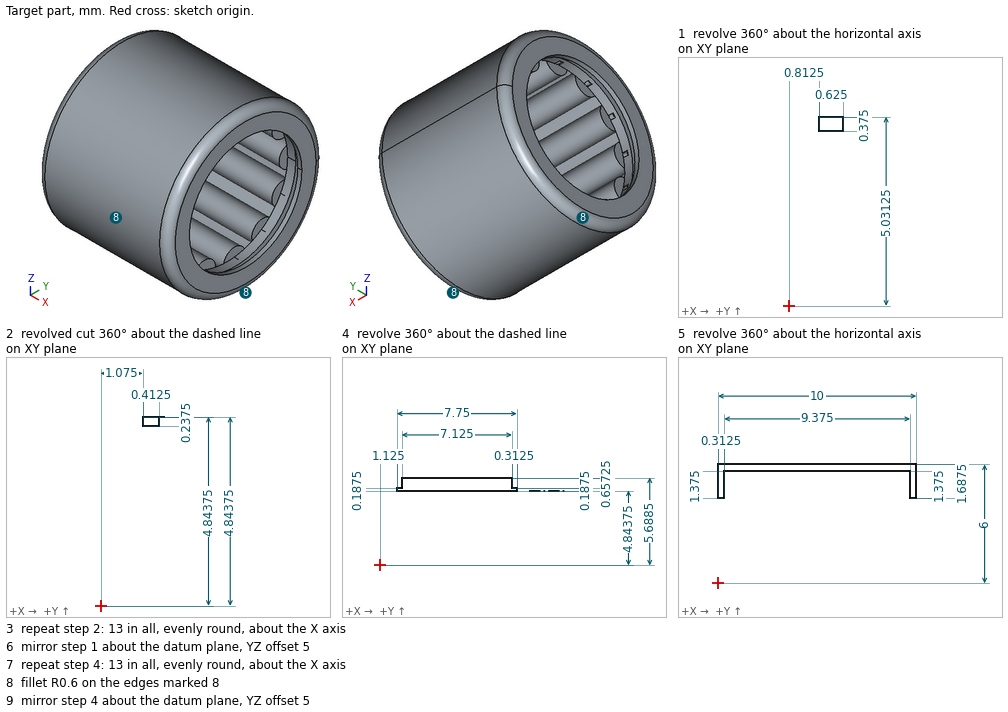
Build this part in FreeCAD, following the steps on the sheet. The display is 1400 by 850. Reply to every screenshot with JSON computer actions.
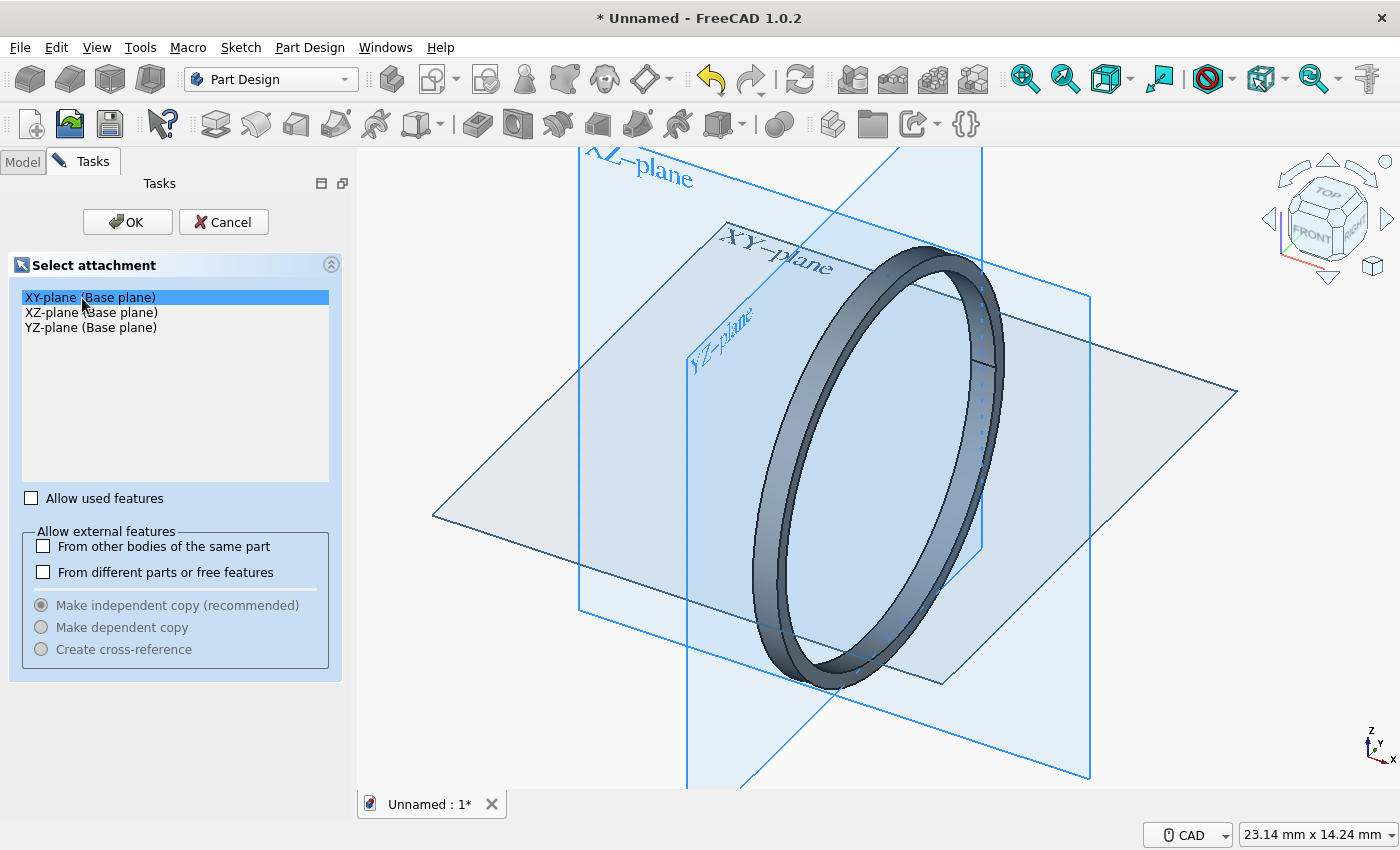
{"action": "left_click", "coordinate": [128, 222]}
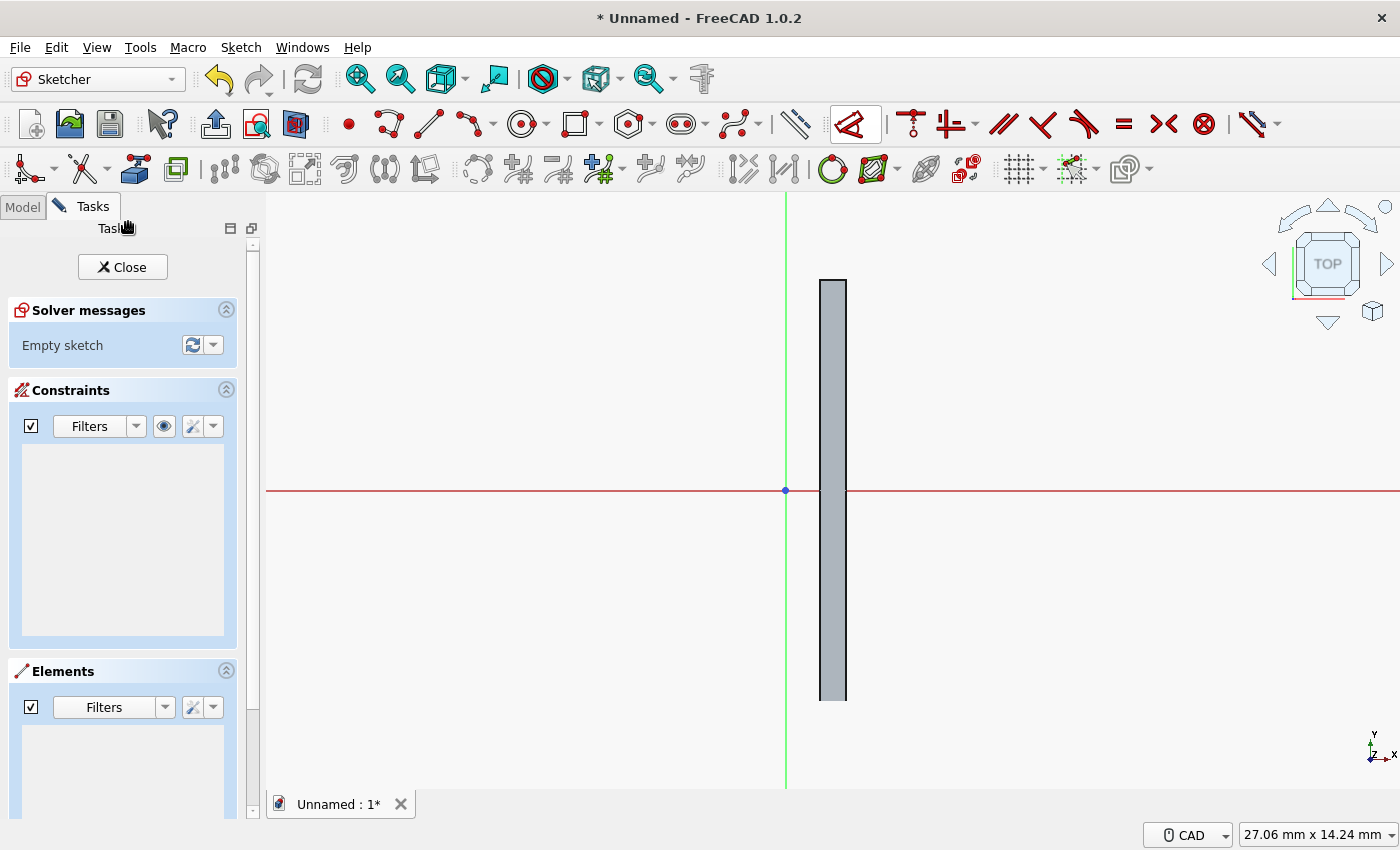
{"action": "key", "text": "q s"}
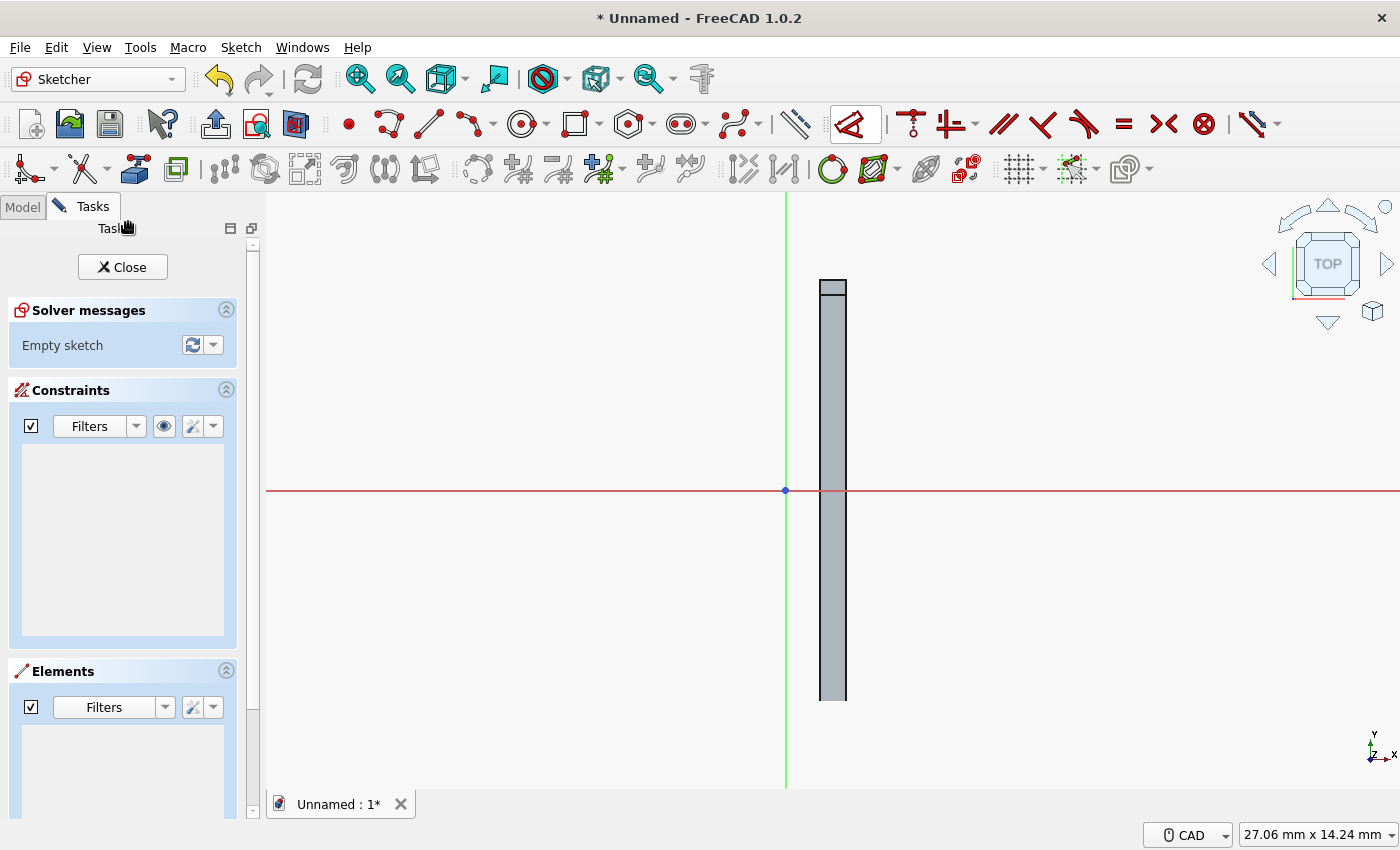
{"action": "scroll", "coordinate": [847, 282], "scroll_direction": "up", "scroll_amount": 15}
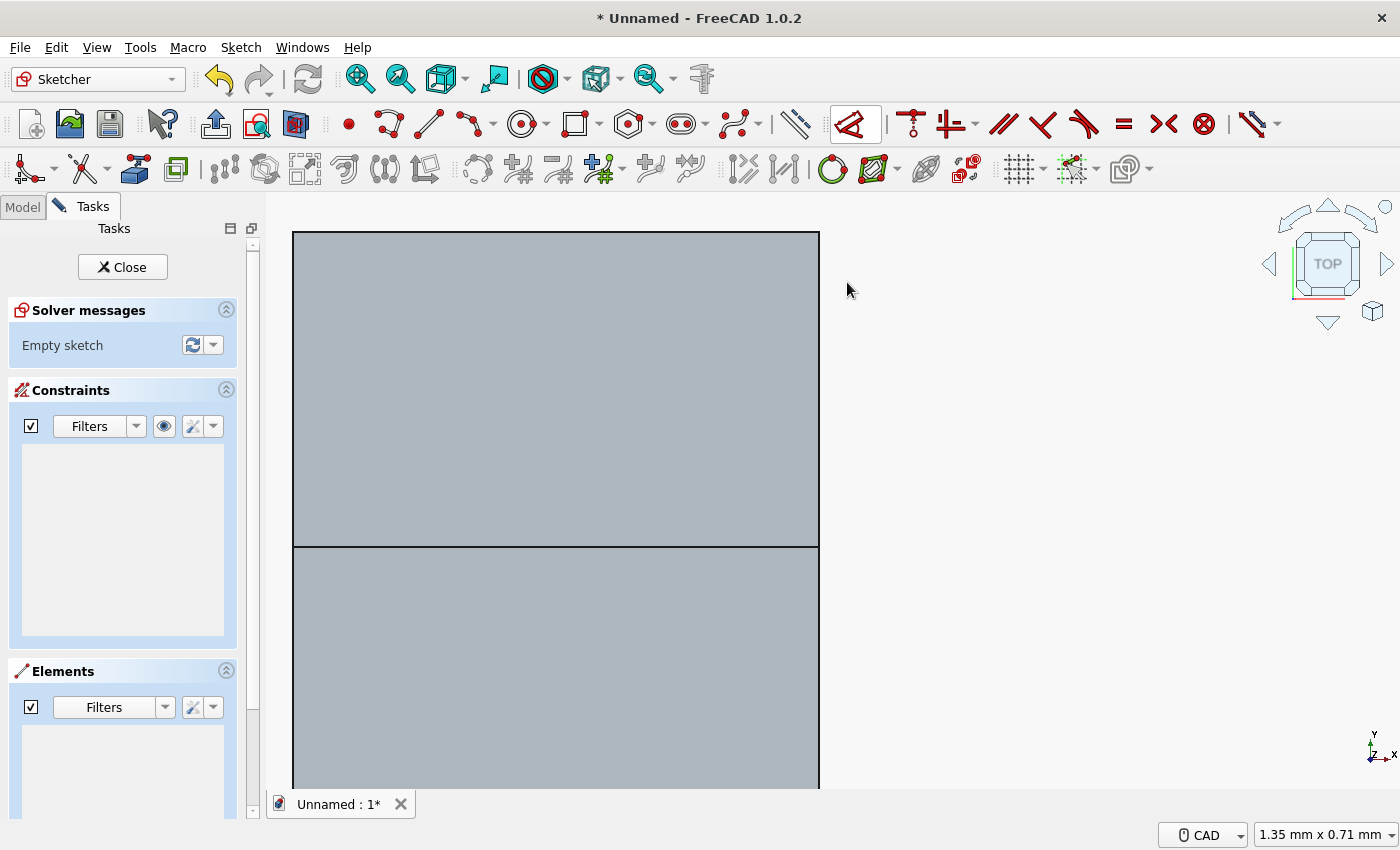
{"action": "scroll", "coordinate": [742, 487], "scroll_direction": "up", "scroll_amount": 2}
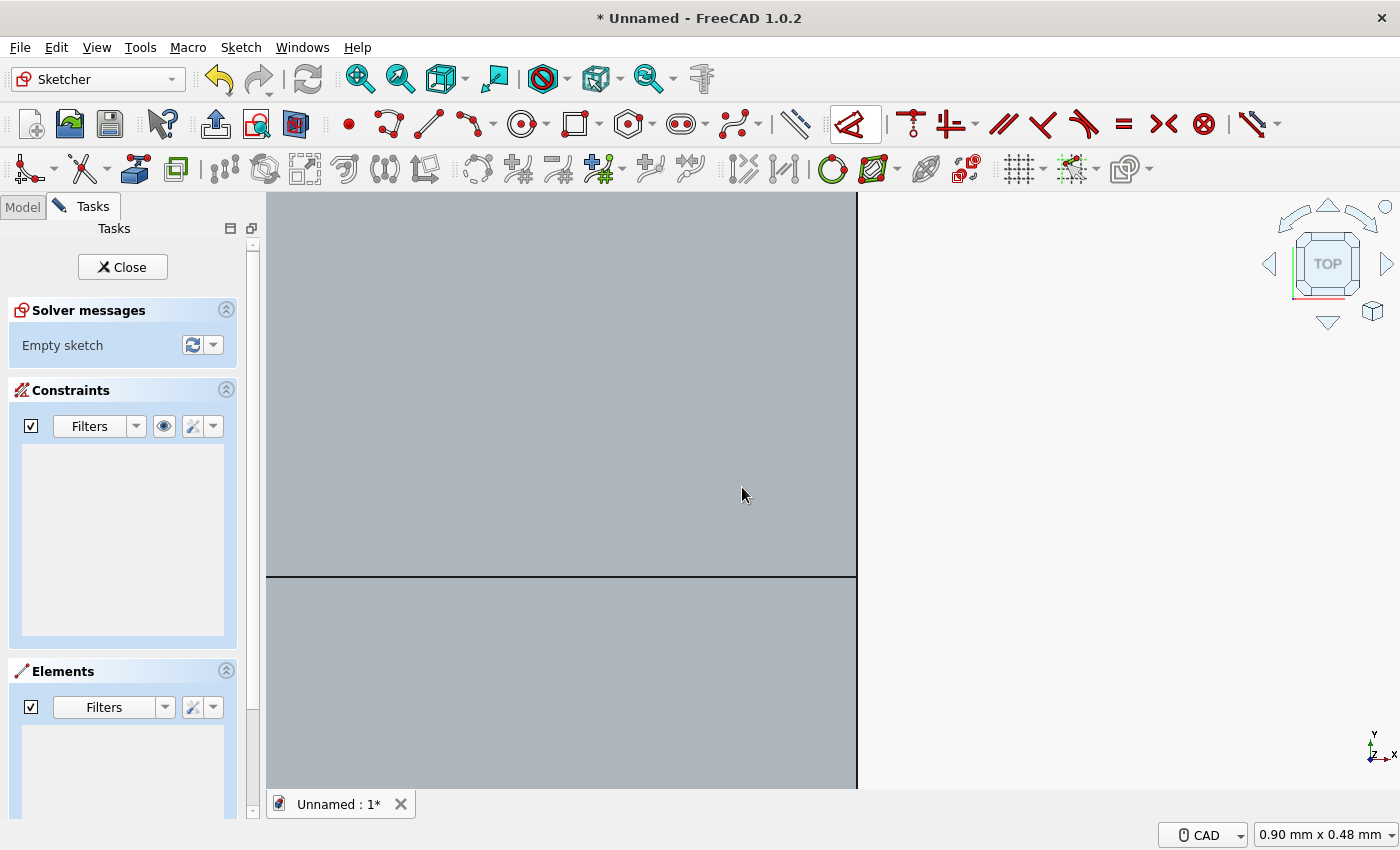
{"action": "key", "text": "g r"}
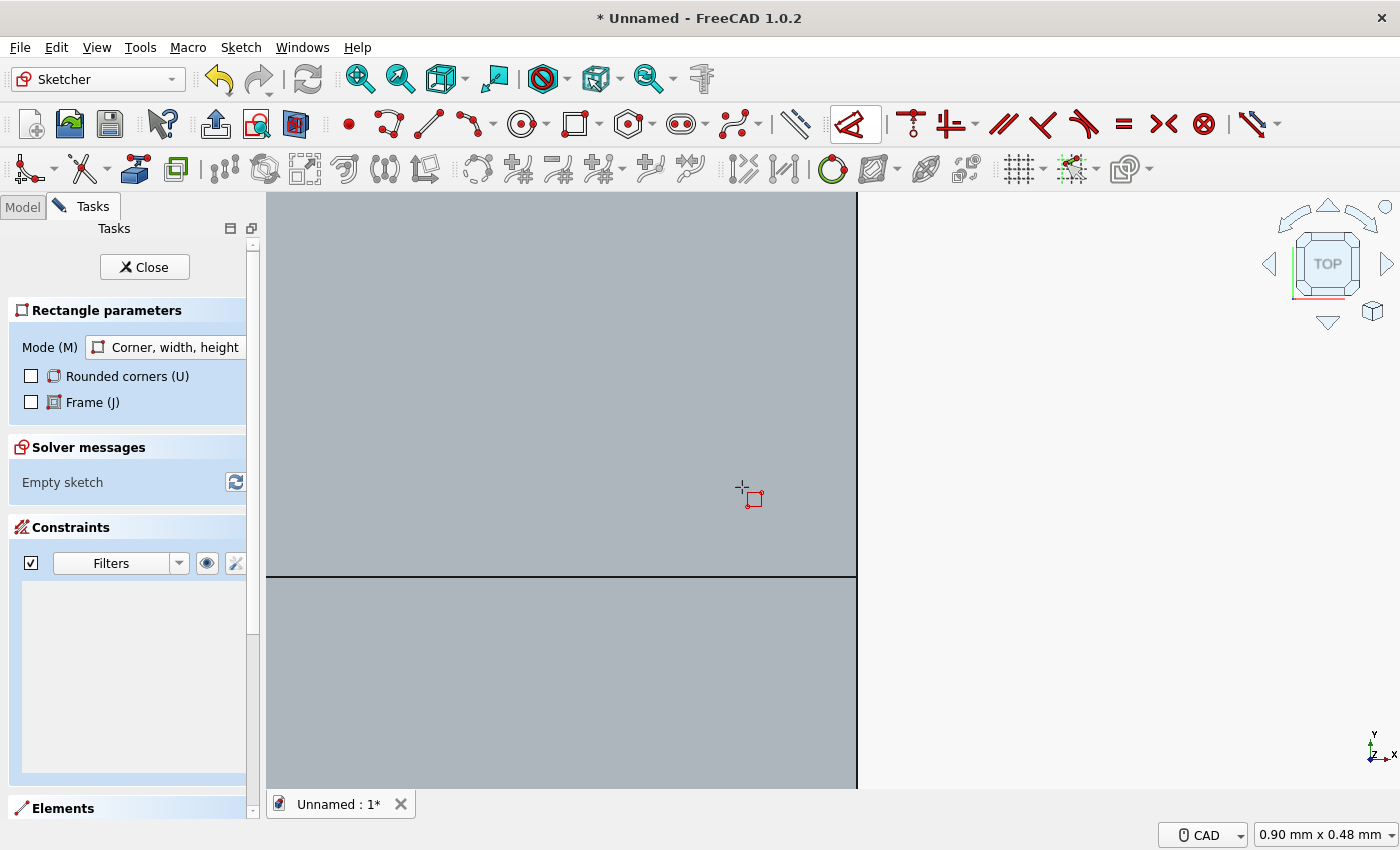
{"action": "left_click", "coordinate": [402, 341]}
{"action": "left_click", "coordinate": [920, 639]}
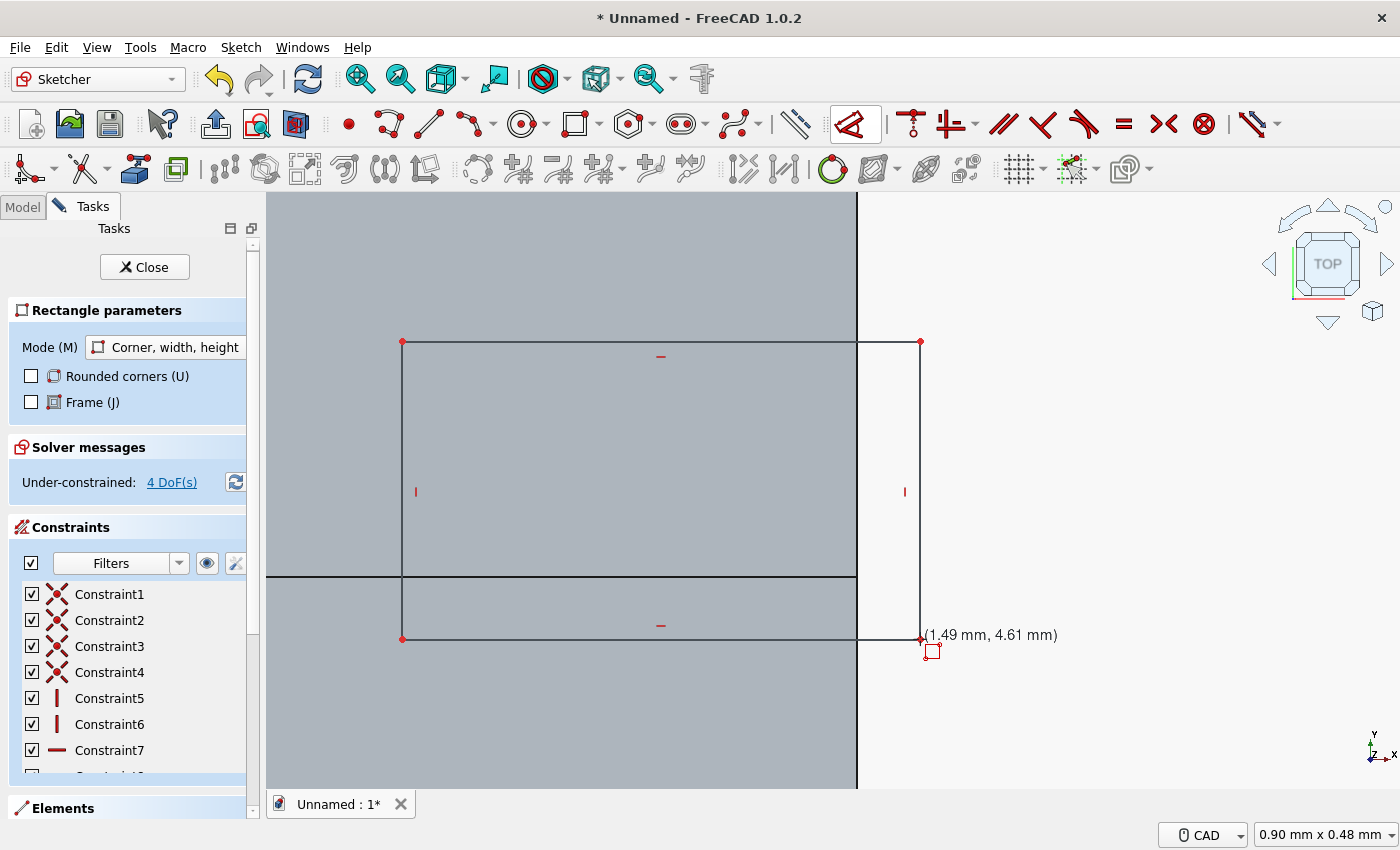
{"action": "key", "text": "g l"}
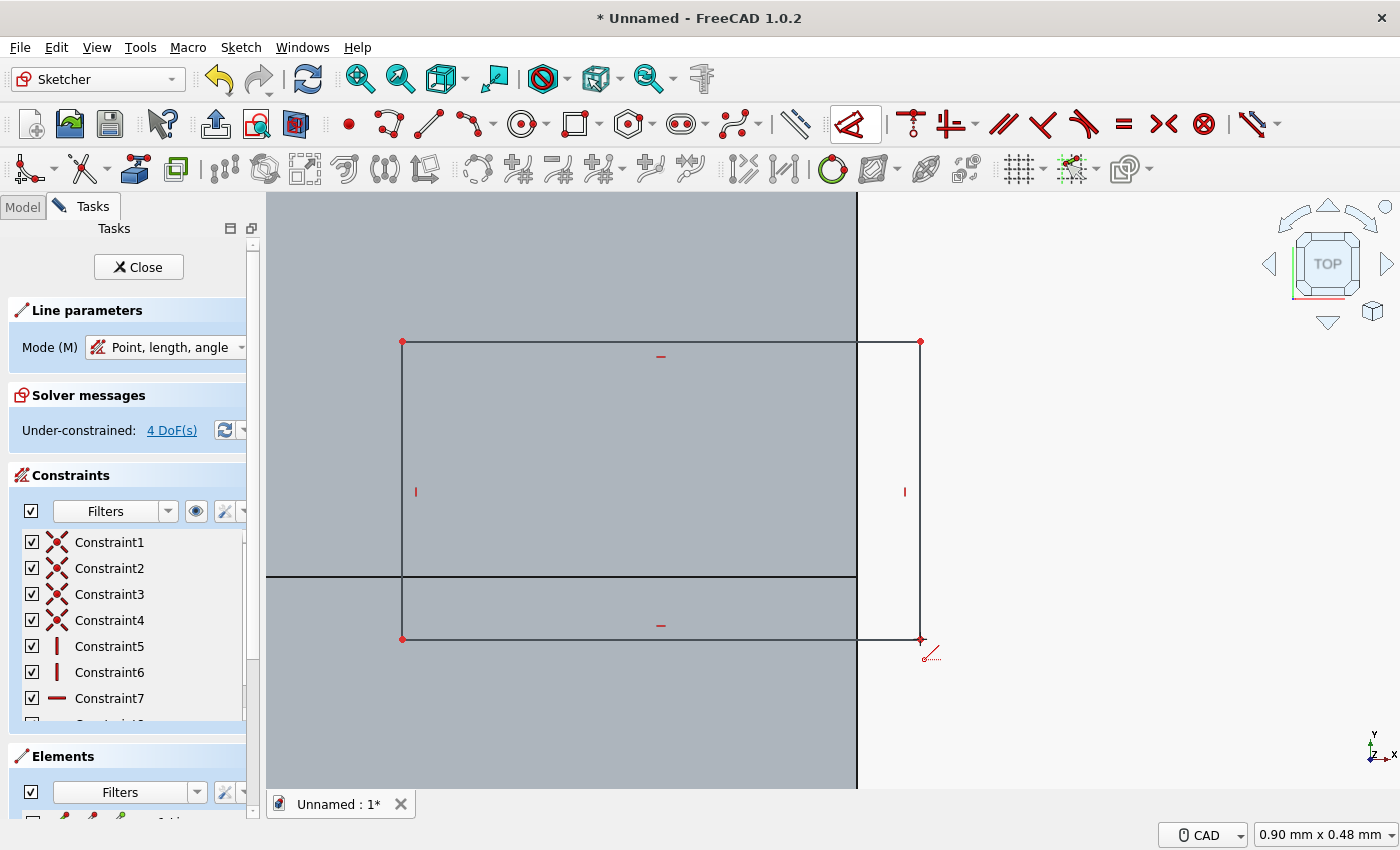
{"action": "left_click", "coordinate": [971, 341]}
{"action": "left_click", "coordinate": [1127, 341]}
{"action": "key", "text": "Escape"}